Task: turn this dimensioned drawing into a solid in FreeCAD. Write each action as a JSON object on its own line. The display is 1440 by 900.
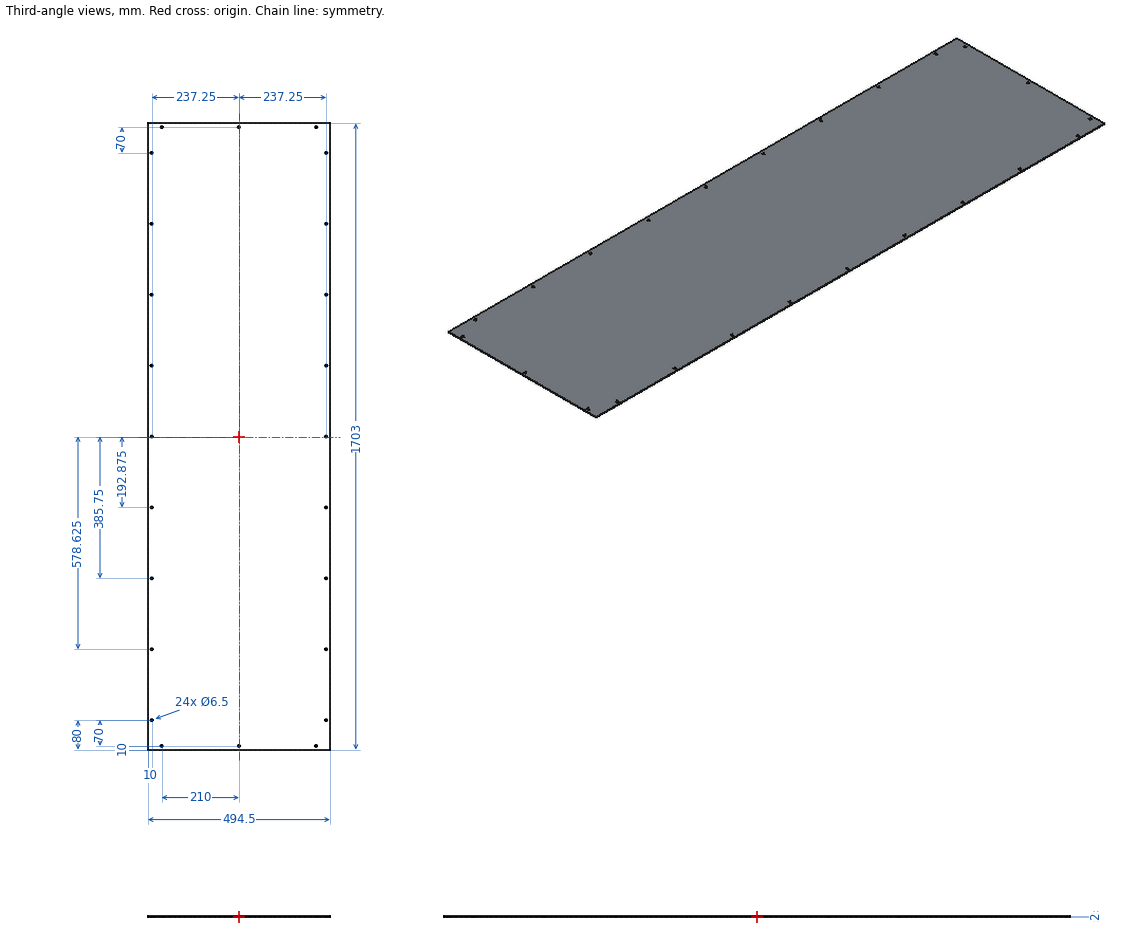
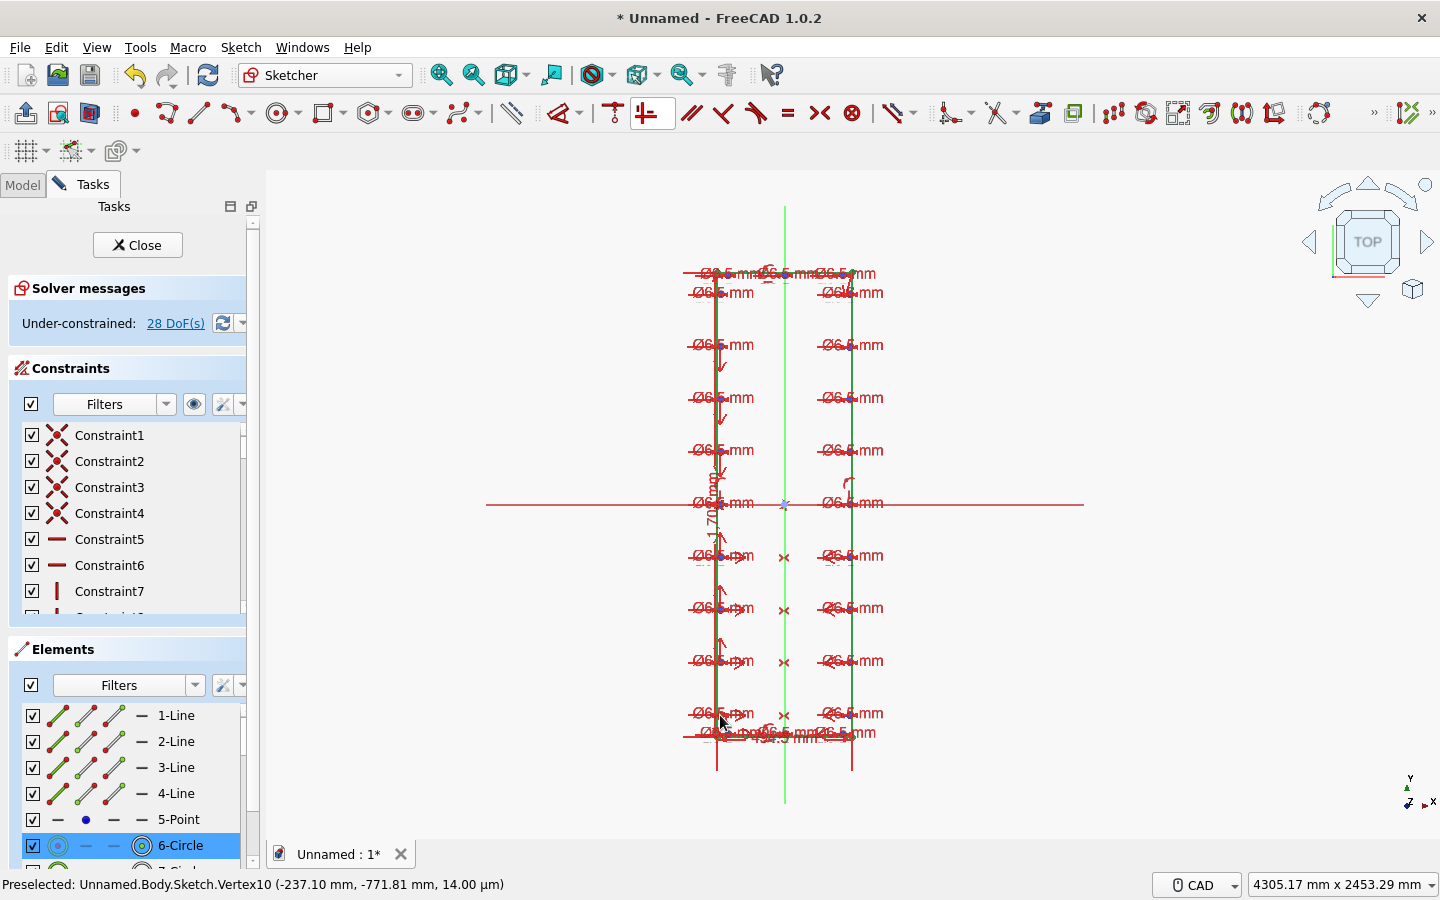
{"action": "left_click", "coordinate": [720, 295]}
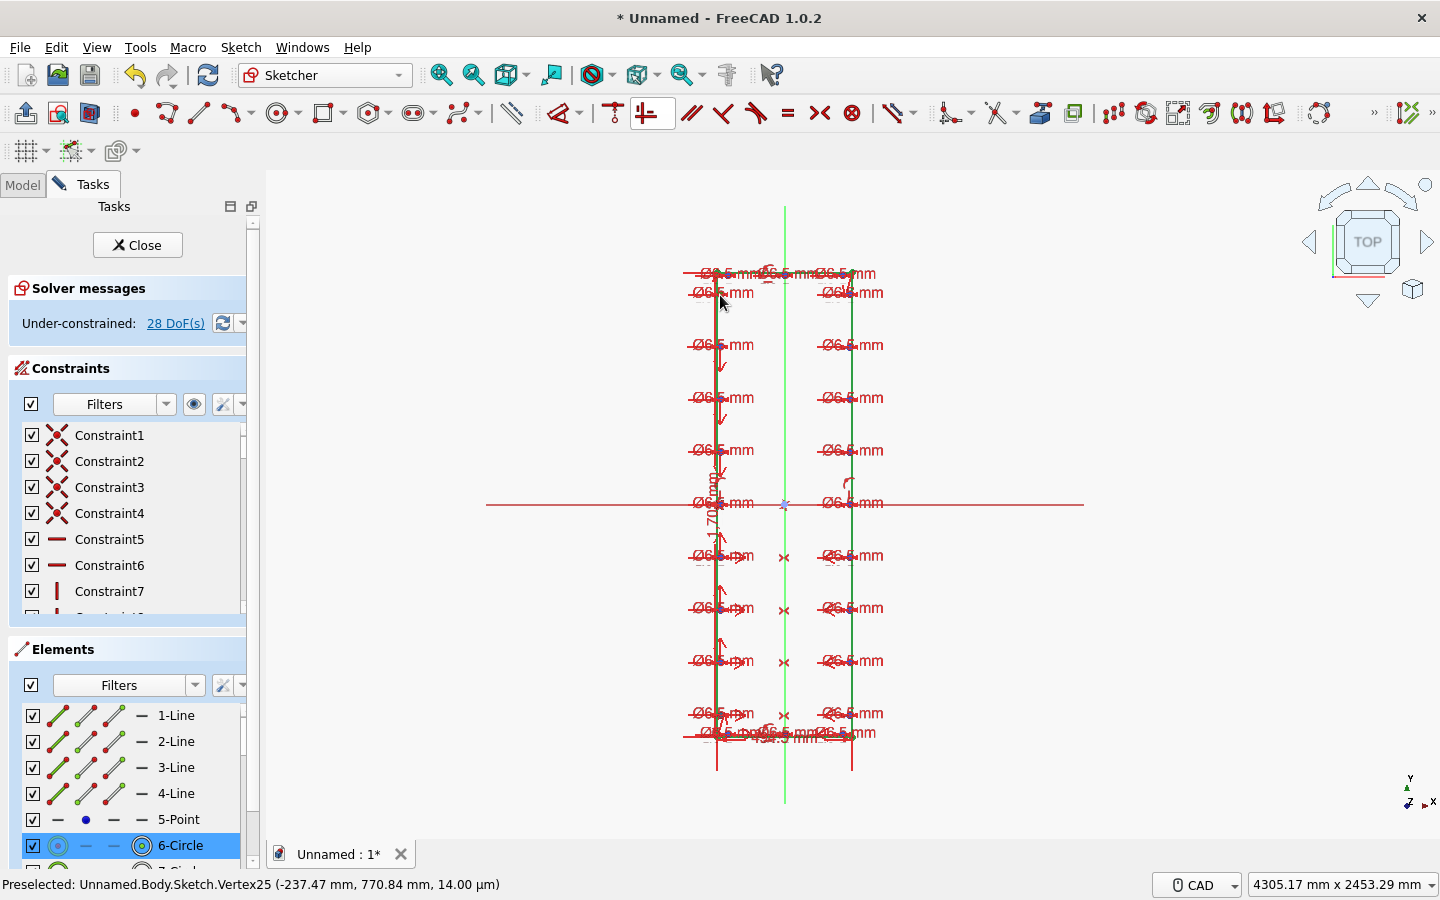
{"action": "left_click", "coordinate": [504, 505]}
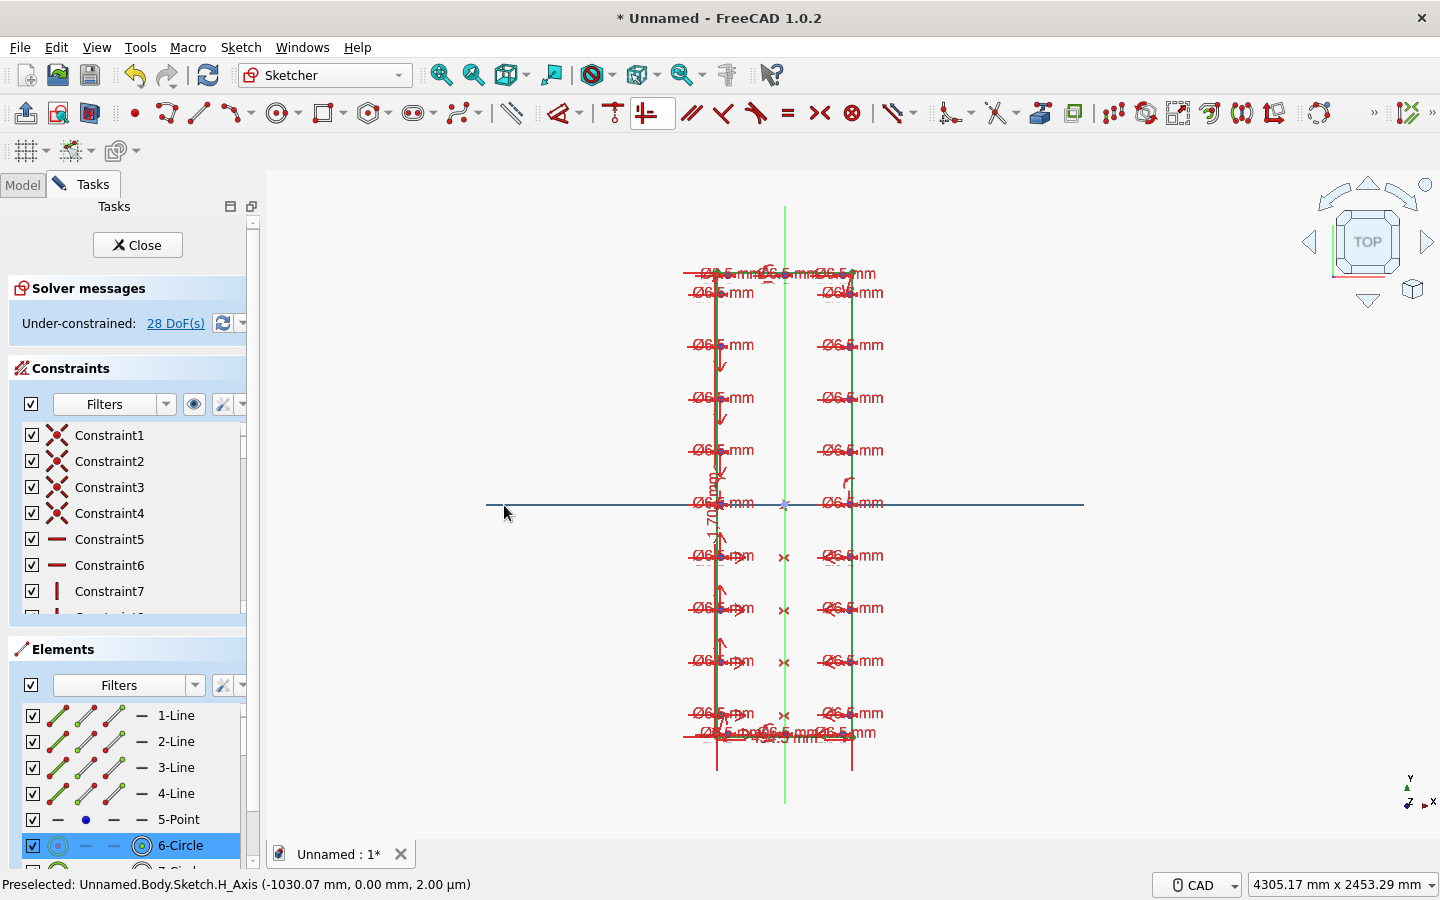
{"action": "left_click", "coordinate": [820, 114]}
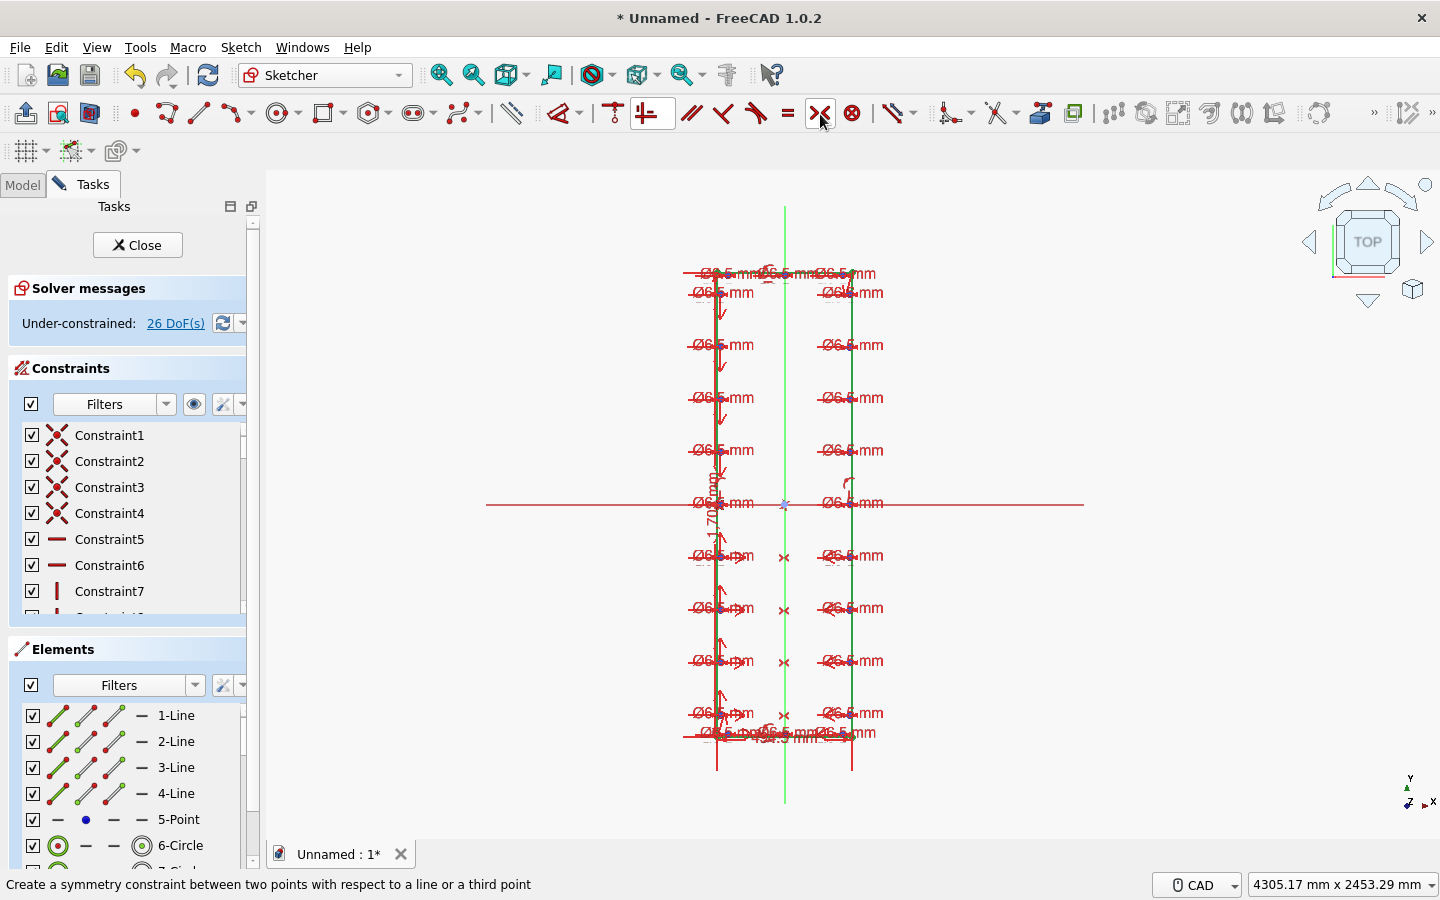
{"action": "left_click", "coordinate": [728, 735]}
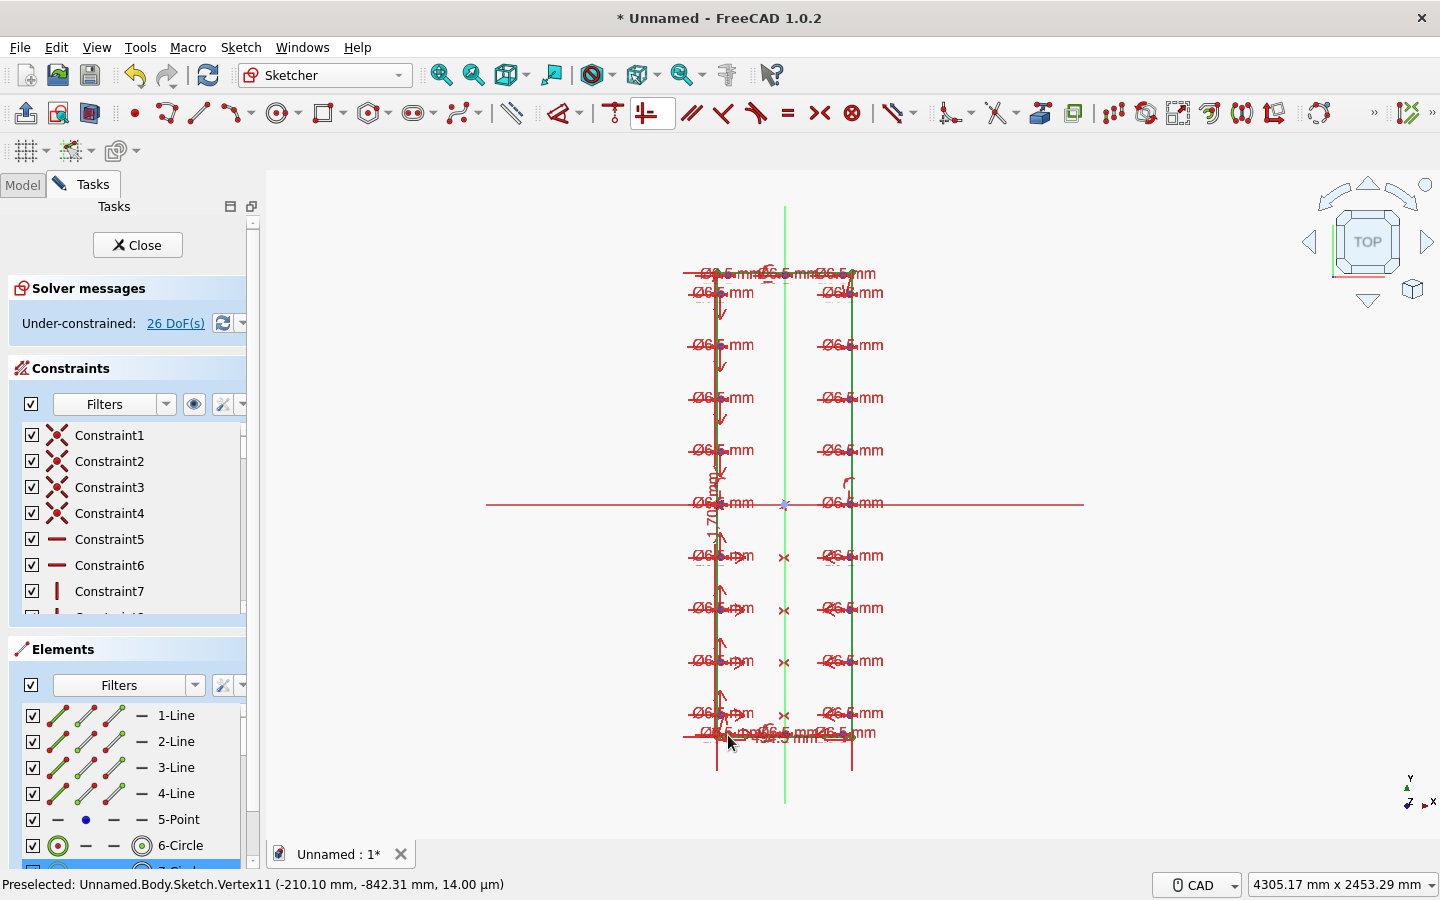
{"action": "left_click", "coordinate": [728, 276]}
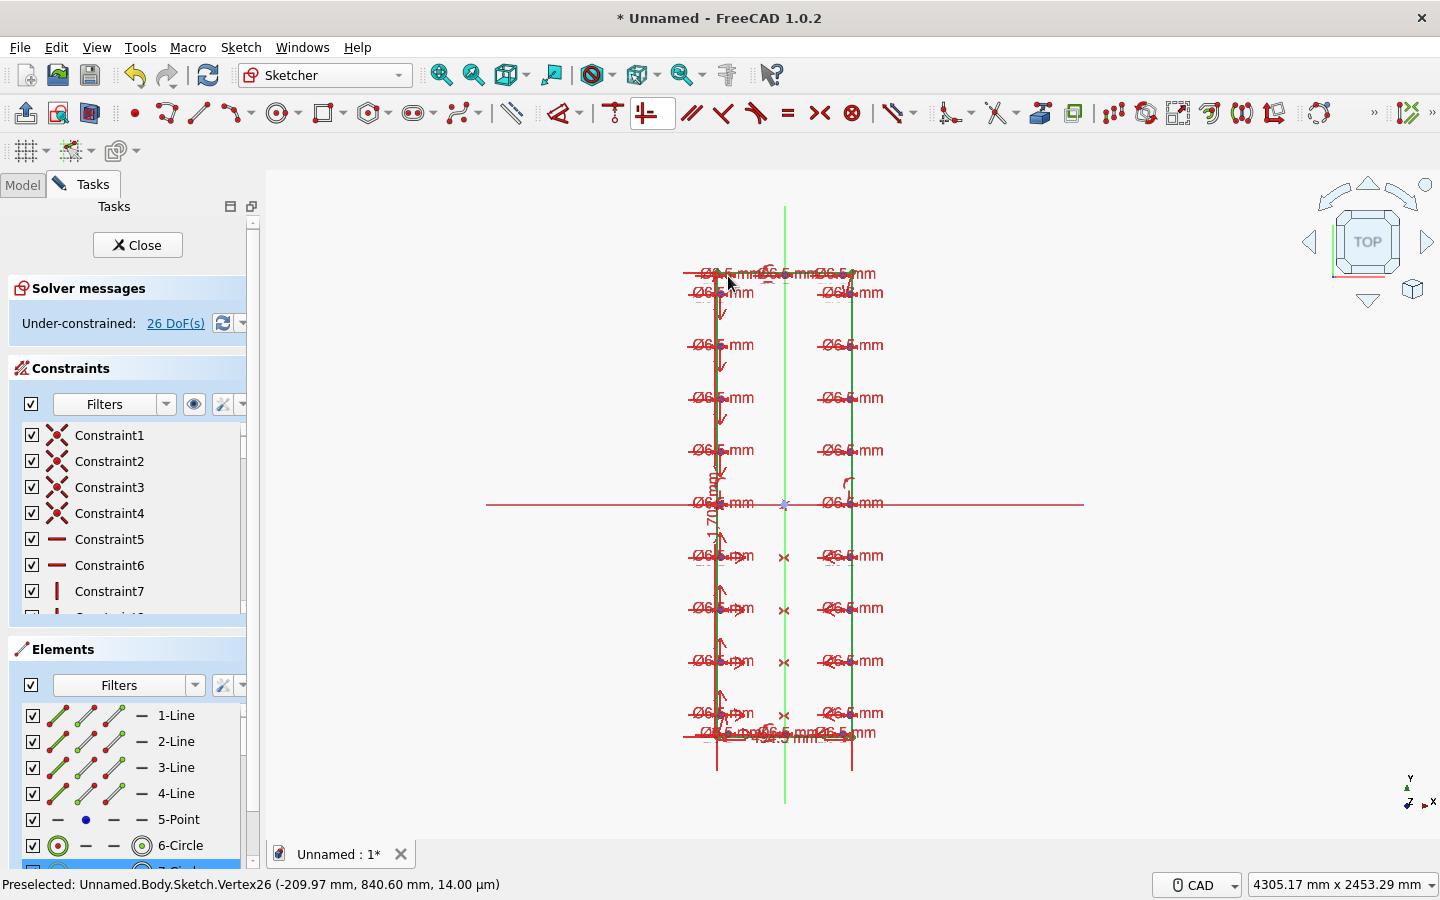
{"action": "left_click", "coordinate": [504, 505]}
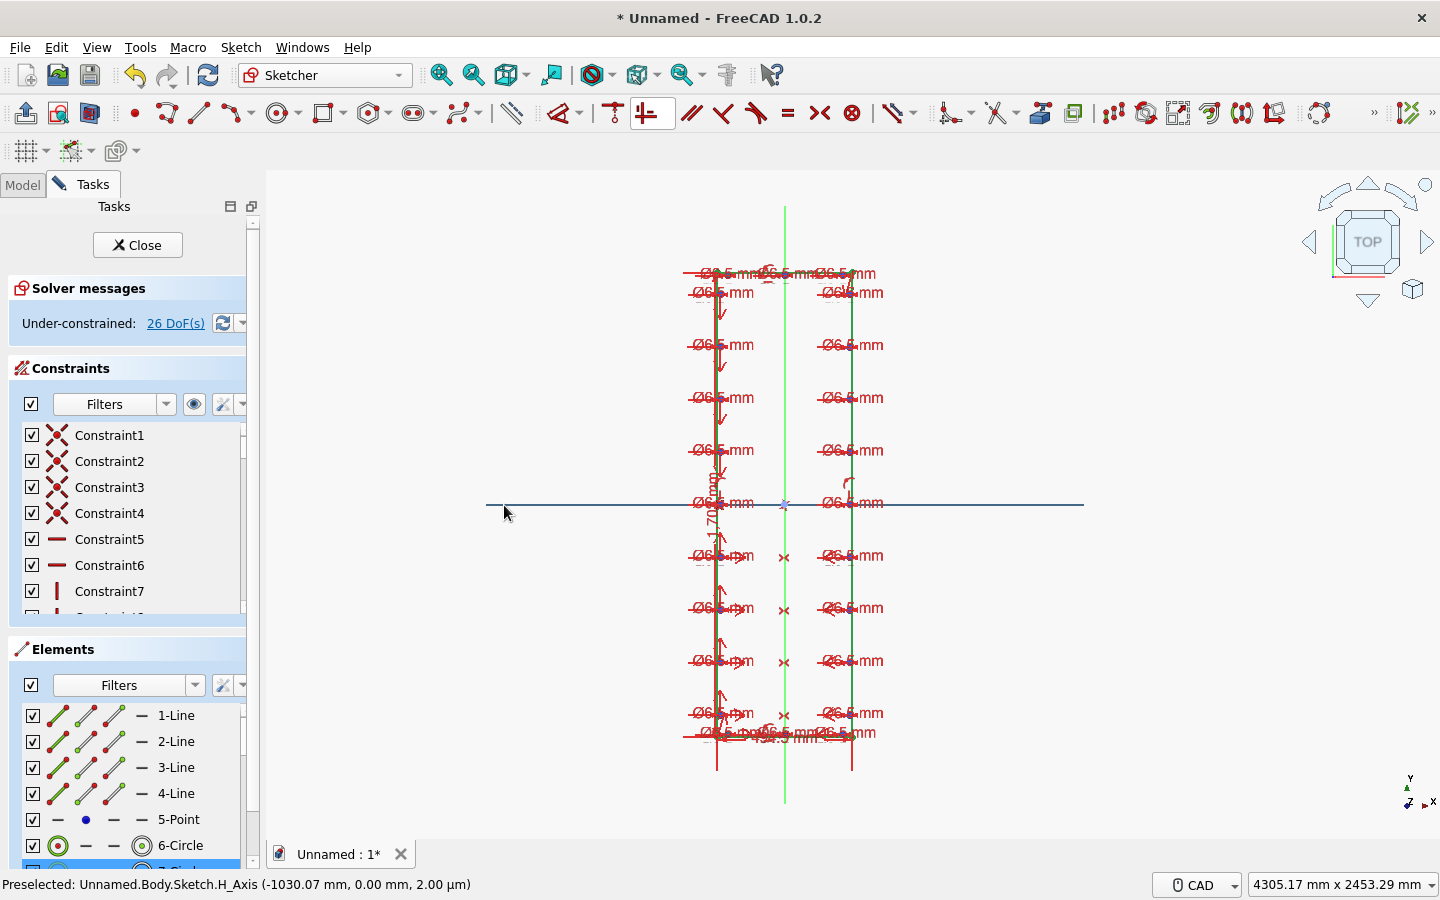
{"action": "left_click", "coordinate": [820, 114]}